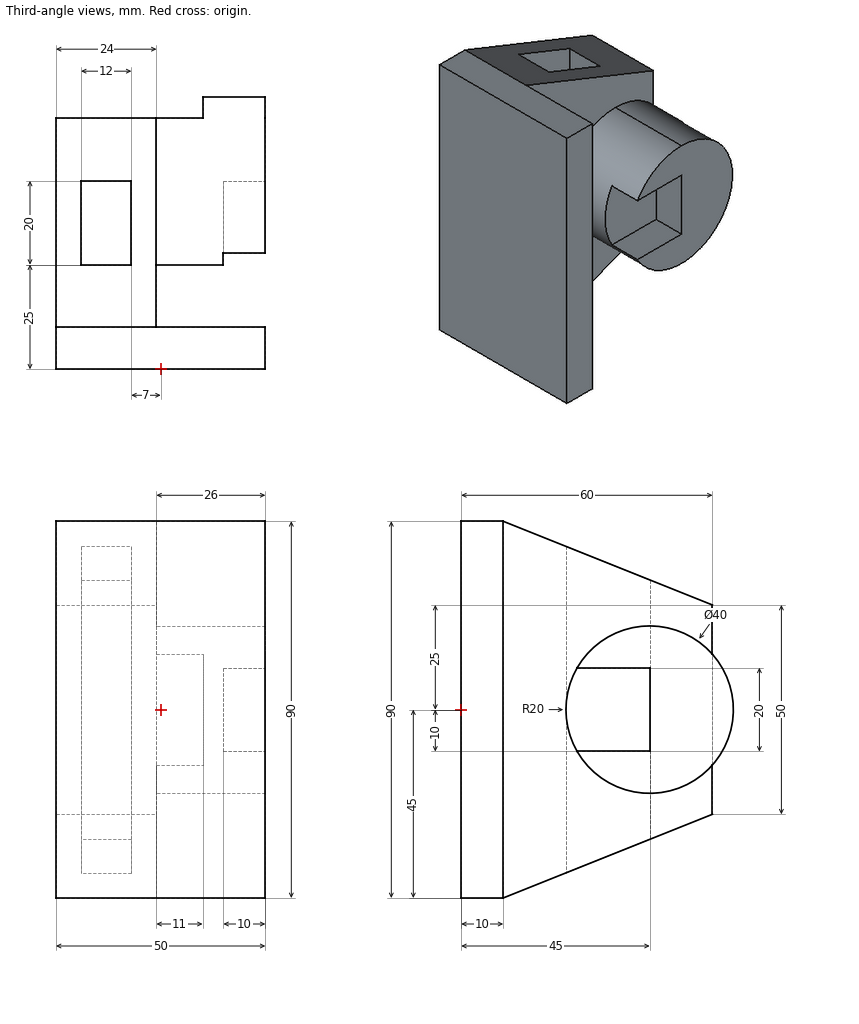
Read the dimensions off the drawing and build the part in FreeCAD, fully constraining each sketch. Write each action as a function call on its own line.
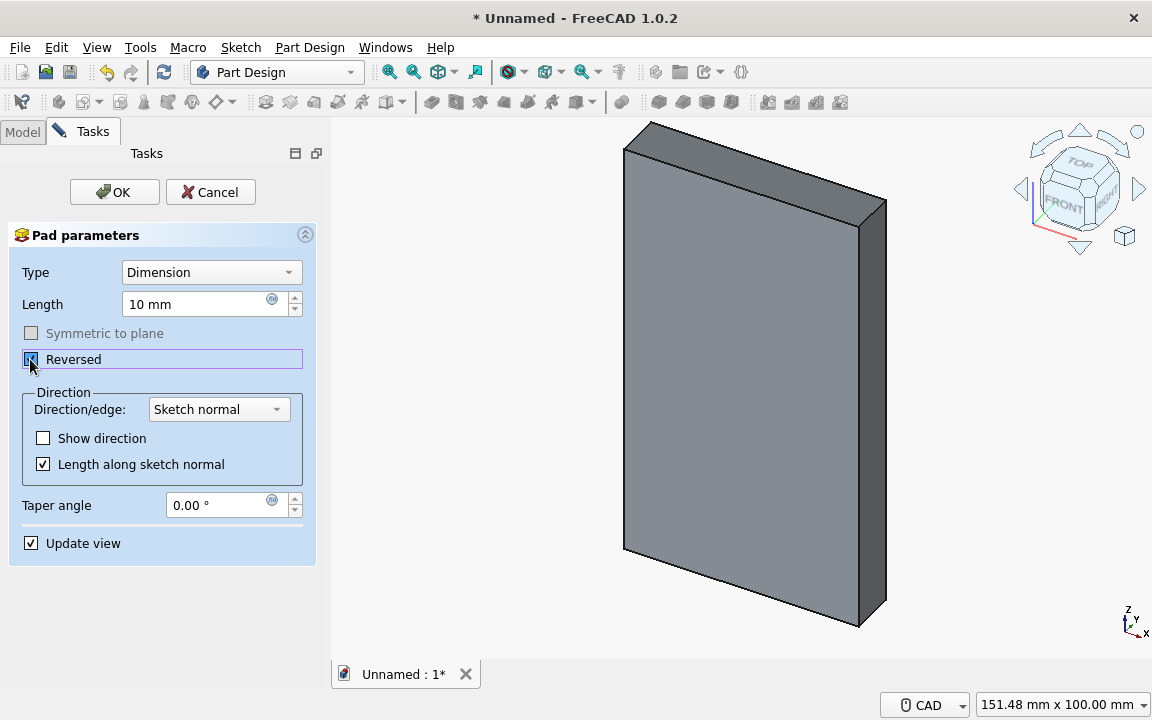
click(115, 192)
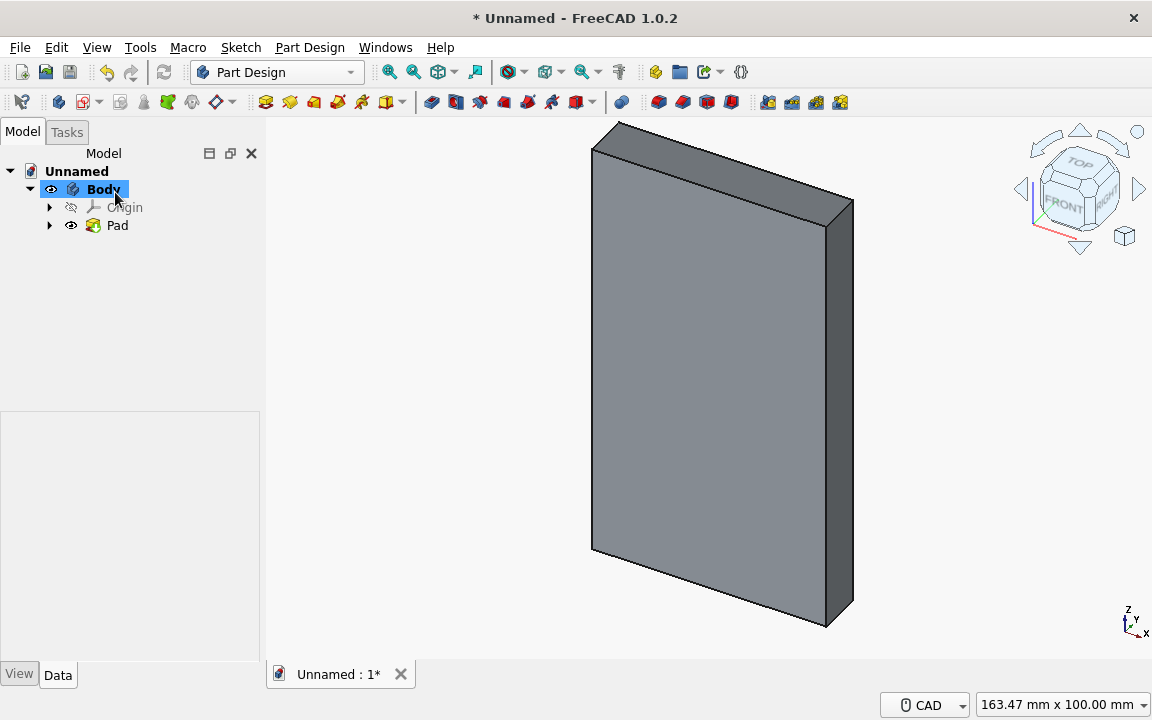
key(6)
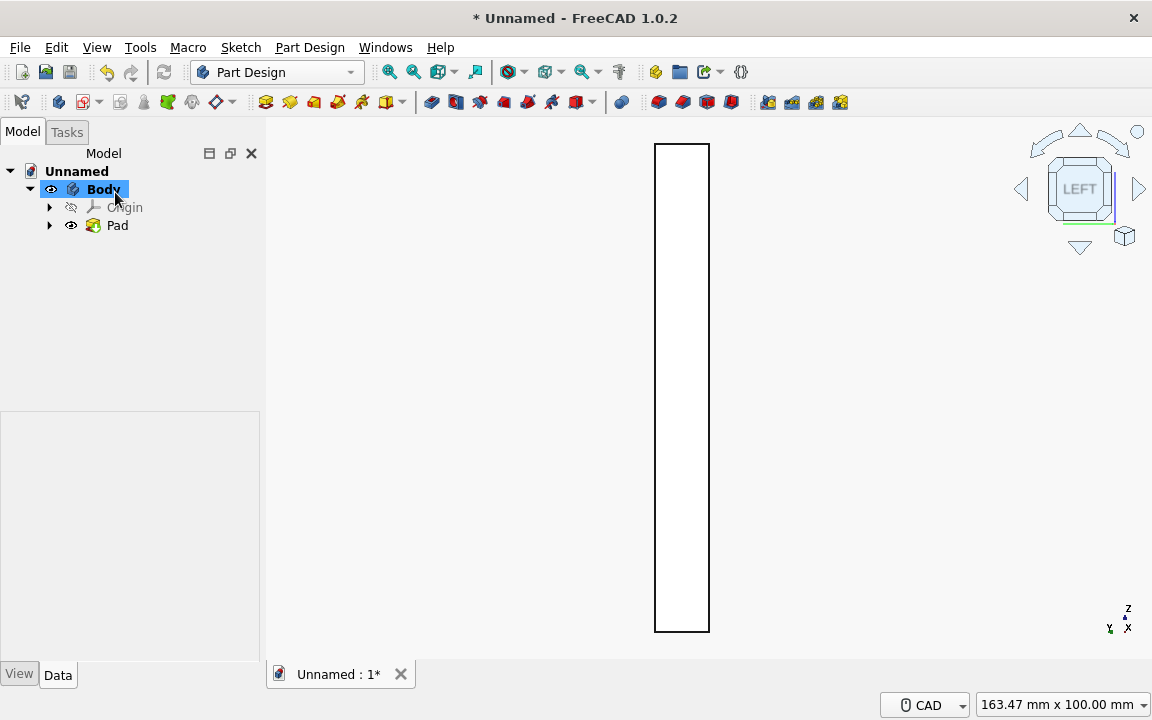
click(682, 178)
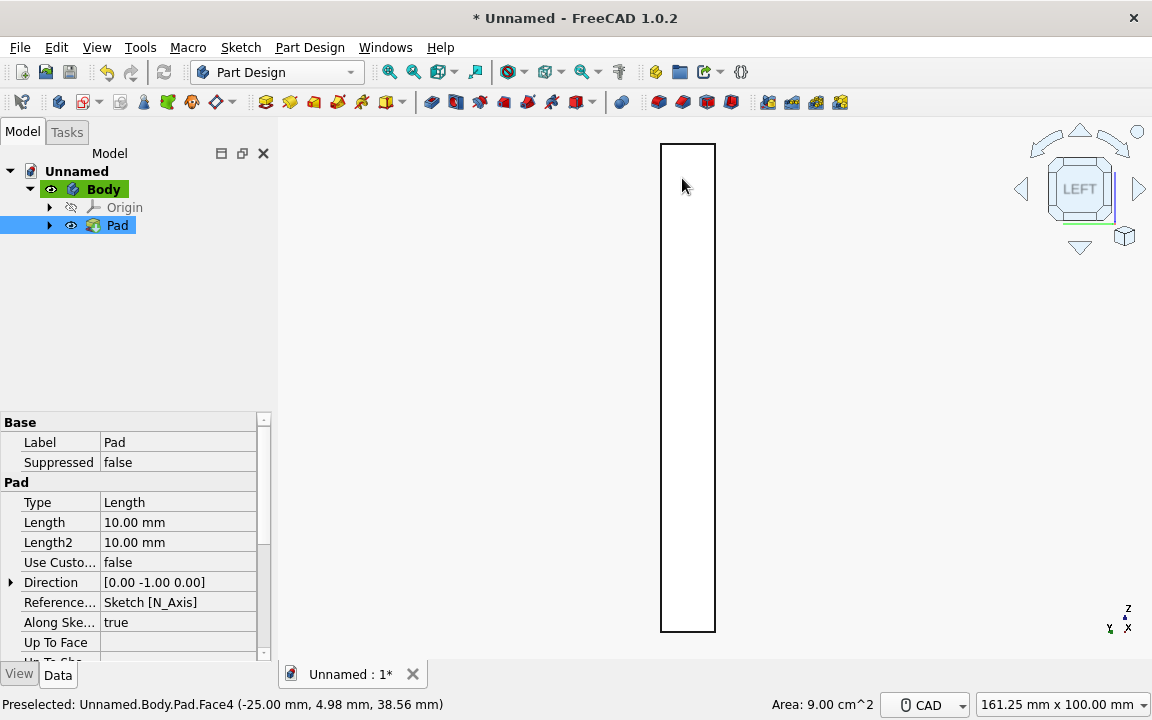
click(84, 102)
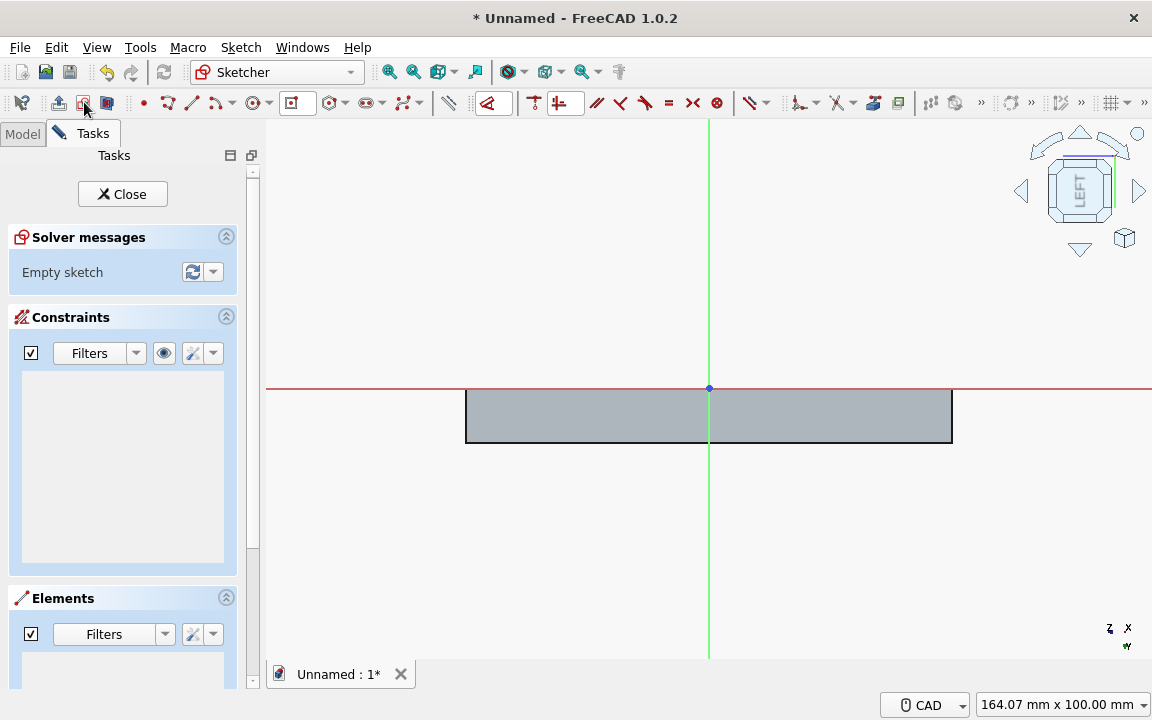
scroll(501, 147, down, 2)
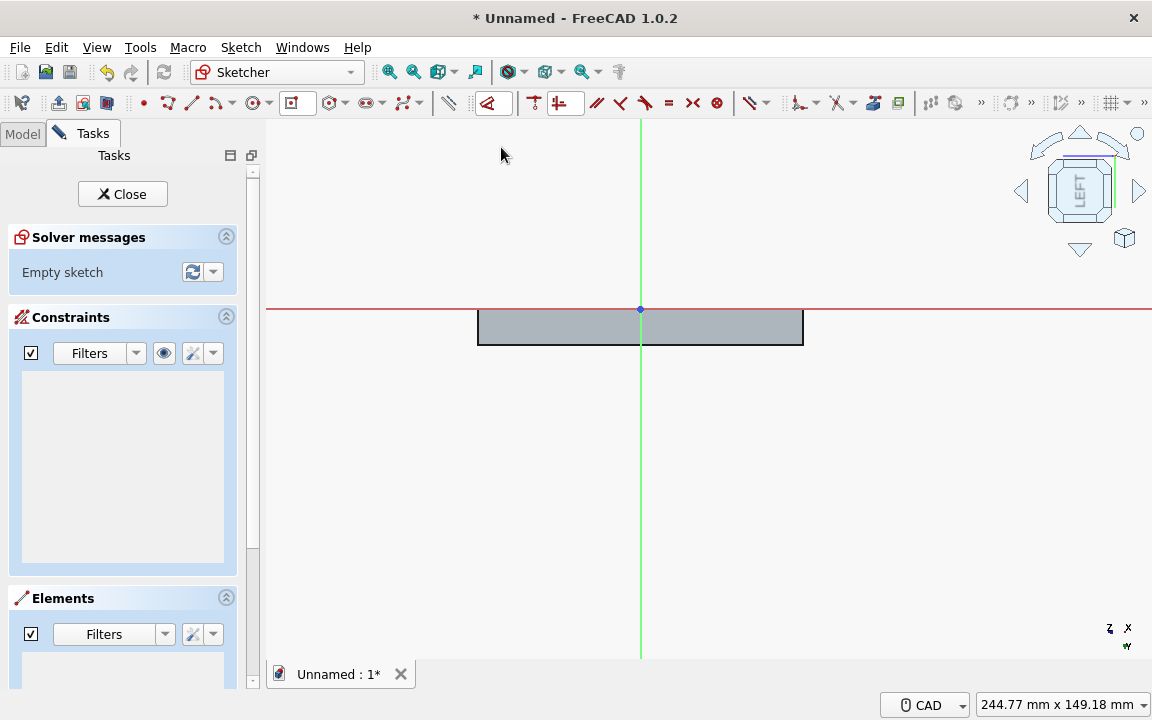
scroll(641, 476, up, 2)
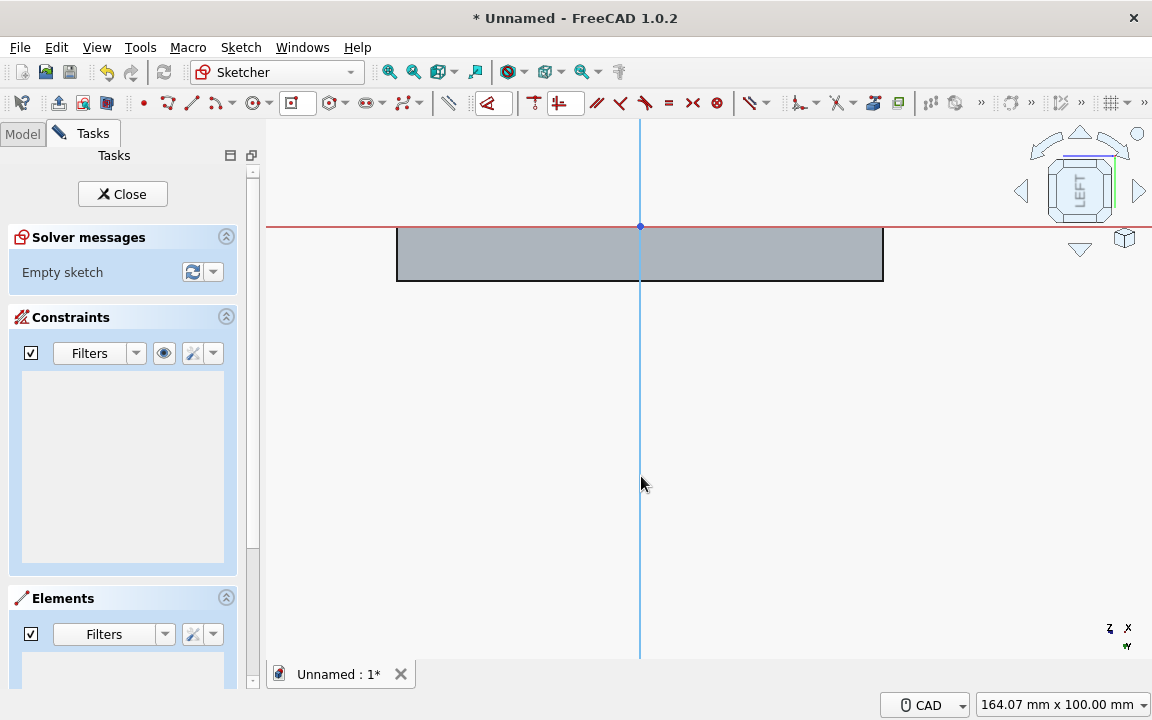
click(168, 104)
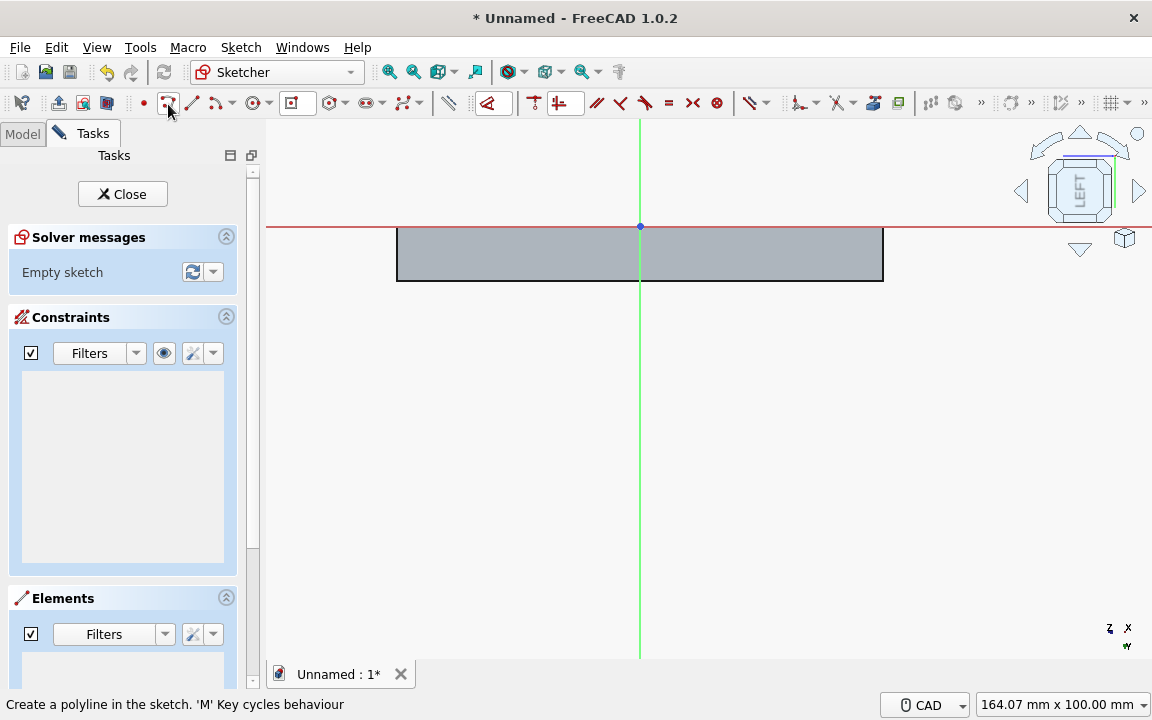
click(883, 281)
click(397, 281)
click(505, 551)
click(775, 551)
click(883, 282)
key(Escape)
key(Escape)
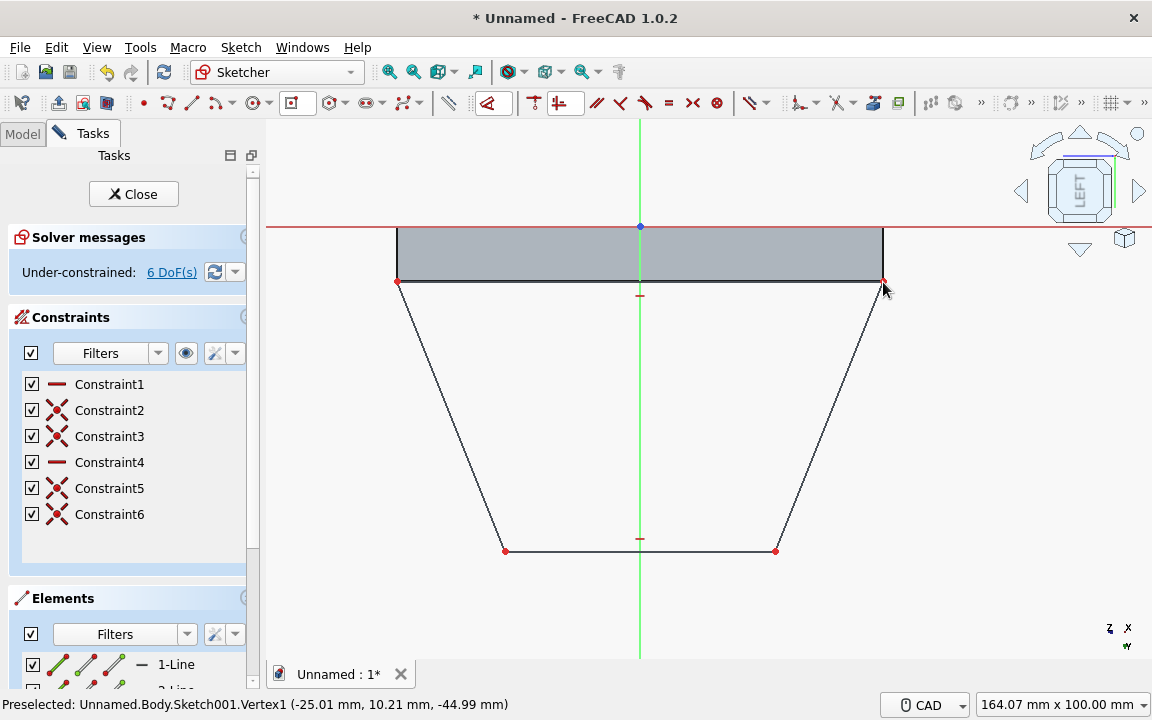
click(488, 104)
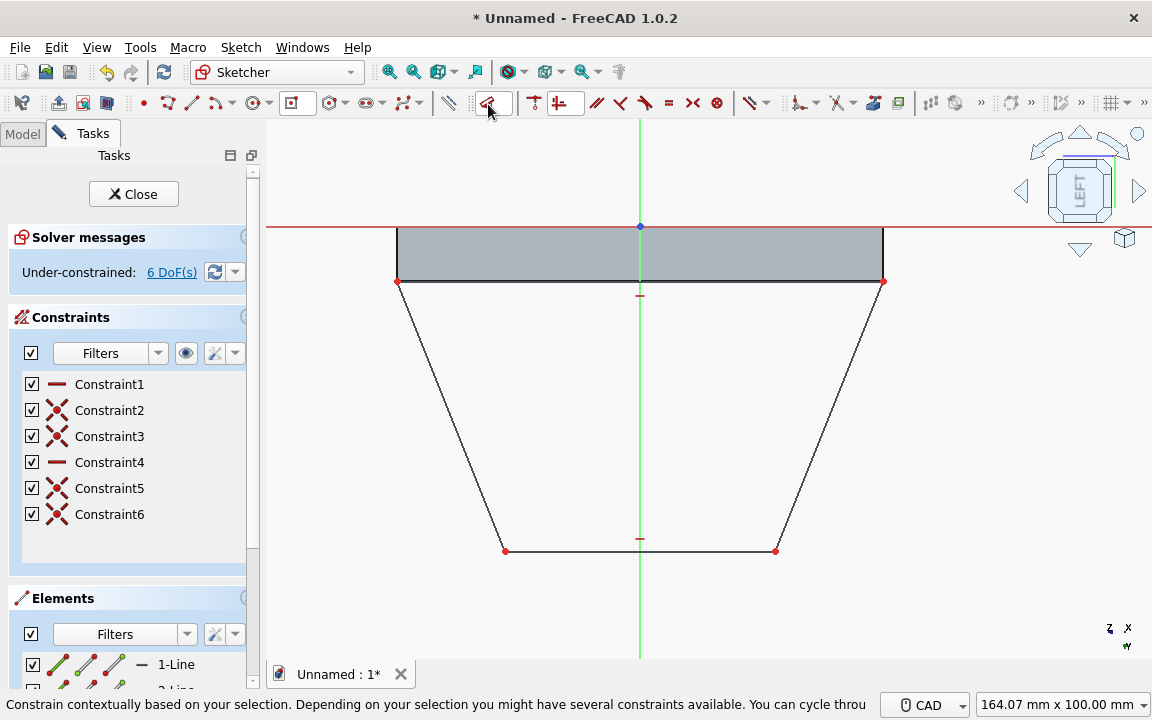
click(737, 282)
click(528, 248)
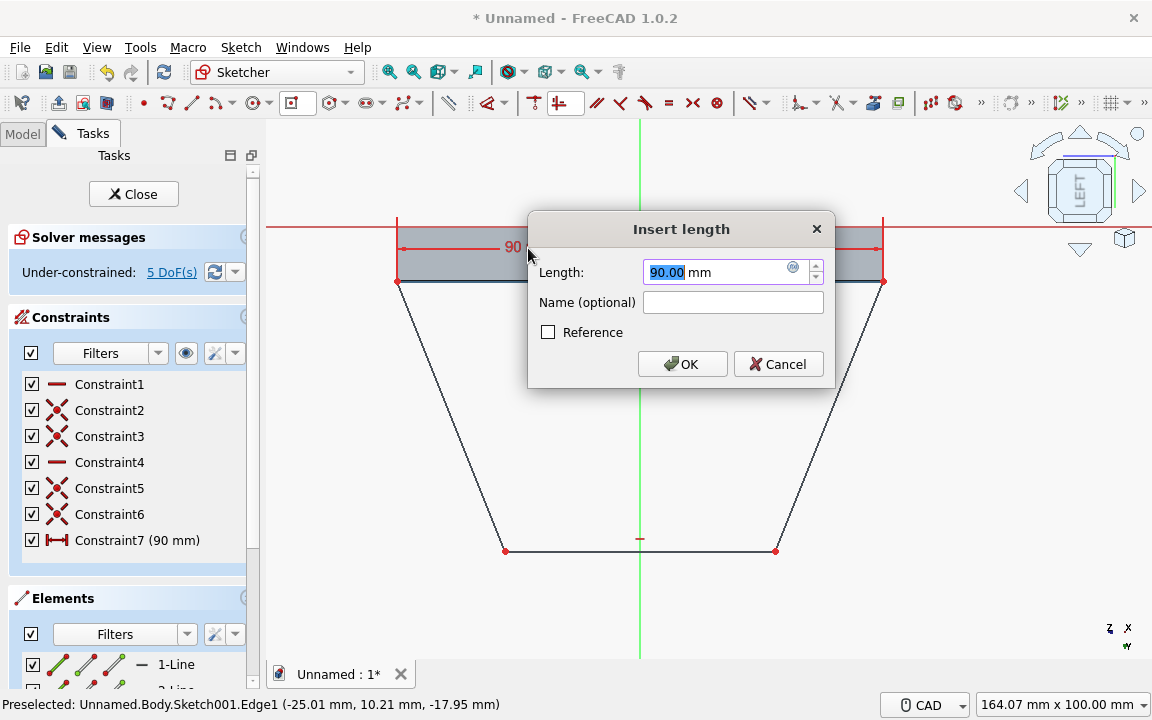
text(90)
key(Return)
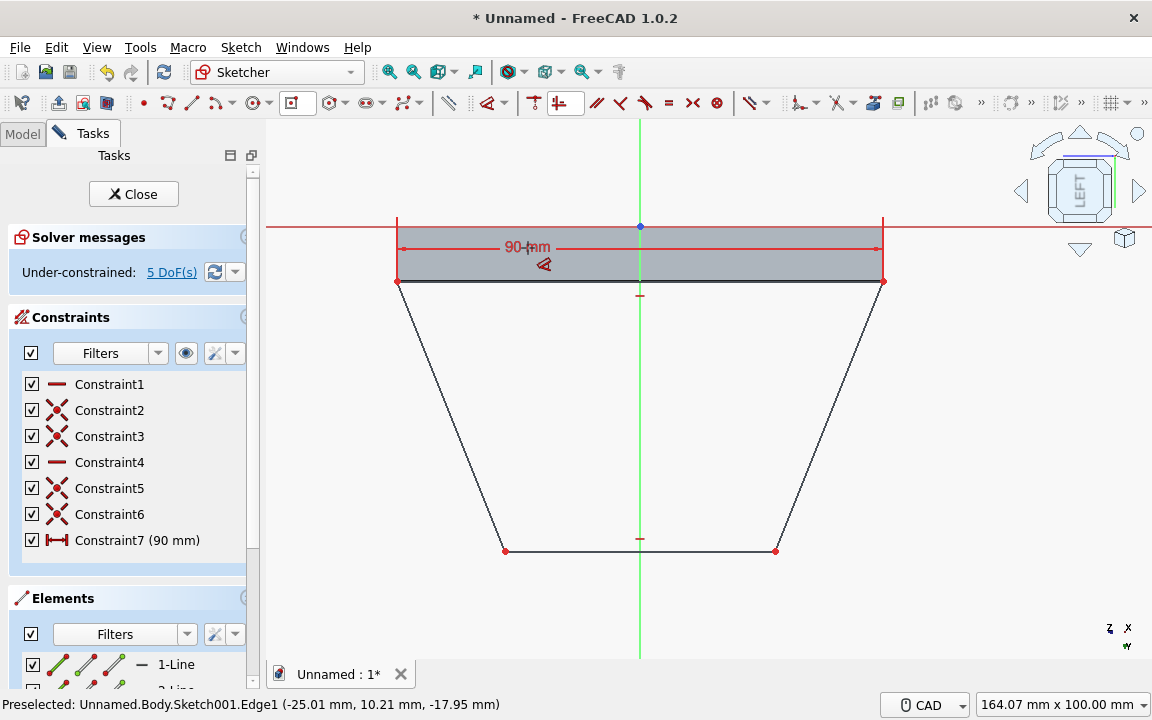
click(586, 552)
click(578, 586)